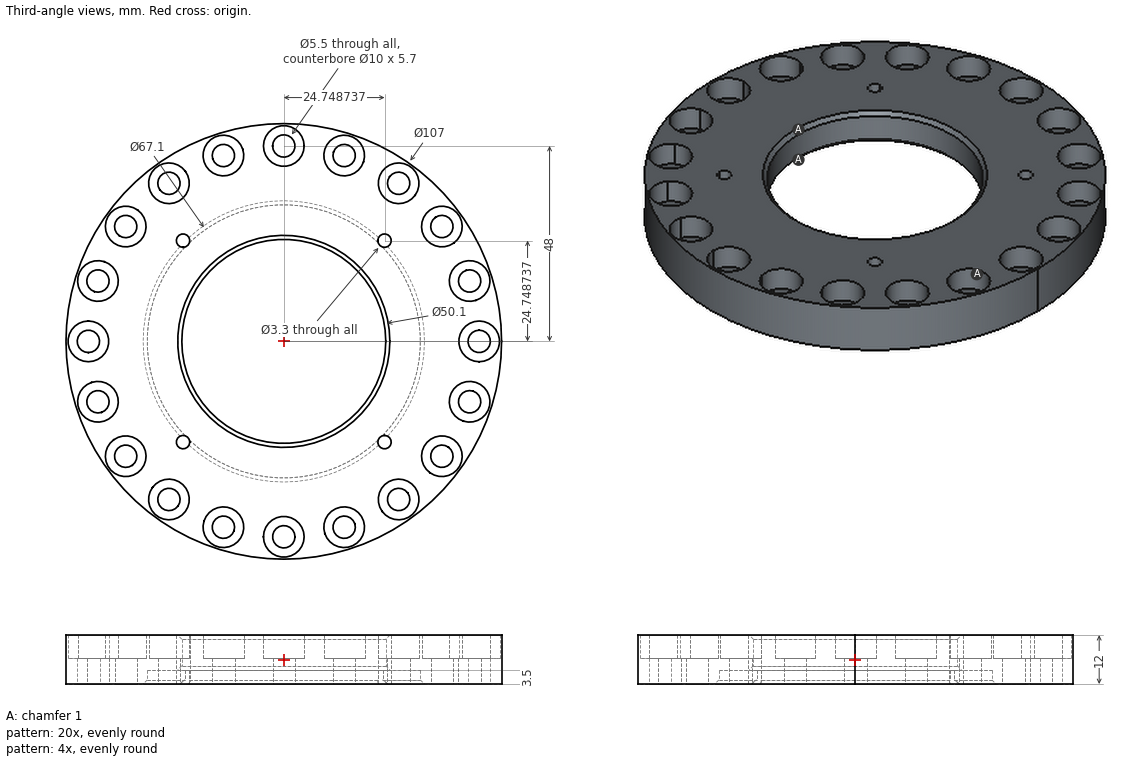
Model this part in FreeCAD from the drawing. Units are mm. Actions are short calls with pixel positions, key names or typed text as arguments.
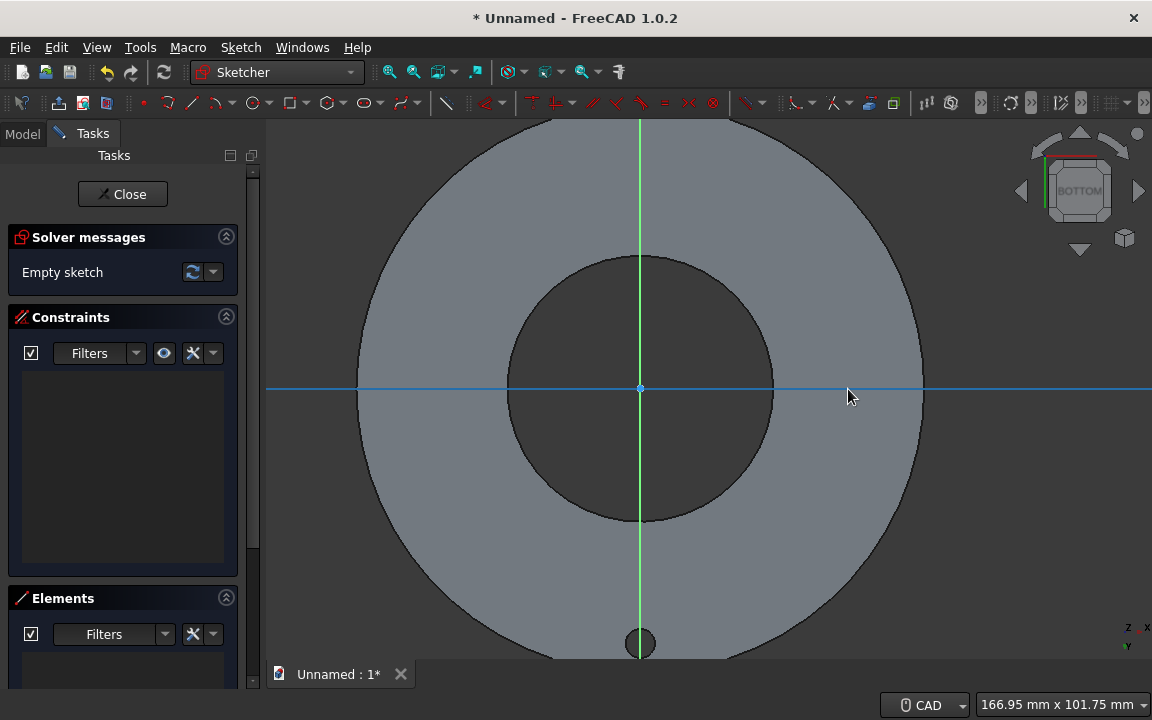
click(254, 104)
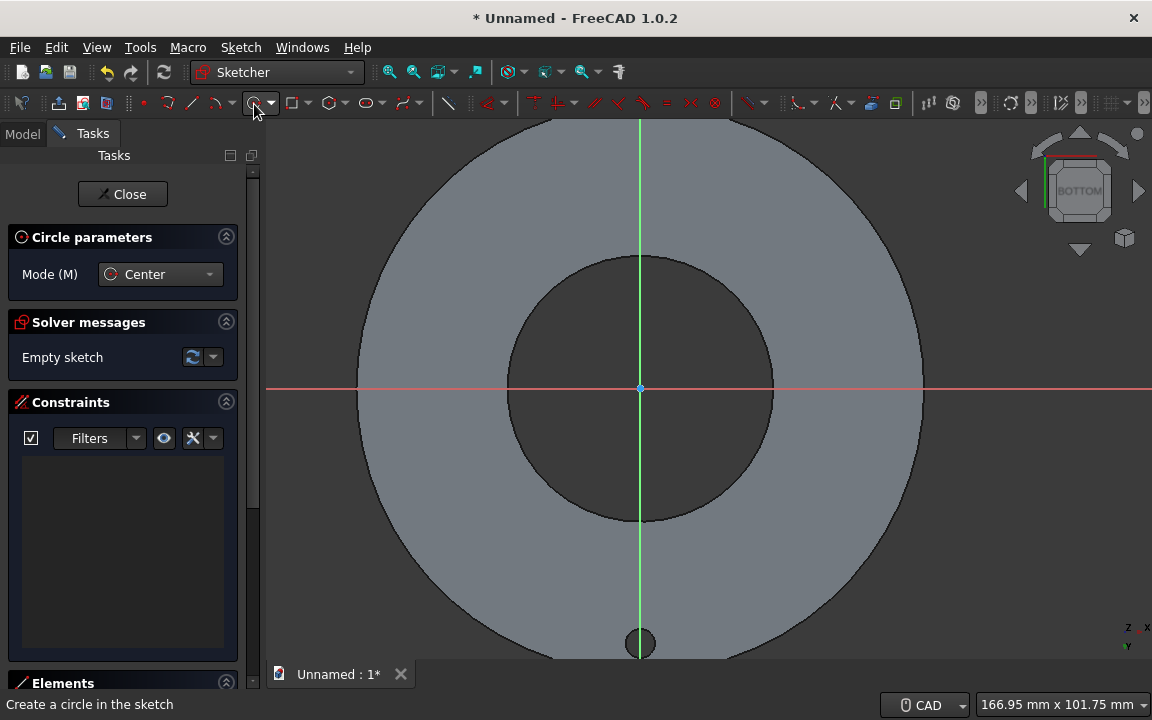
click(640, 389)
click(766, 263)
key(Escape)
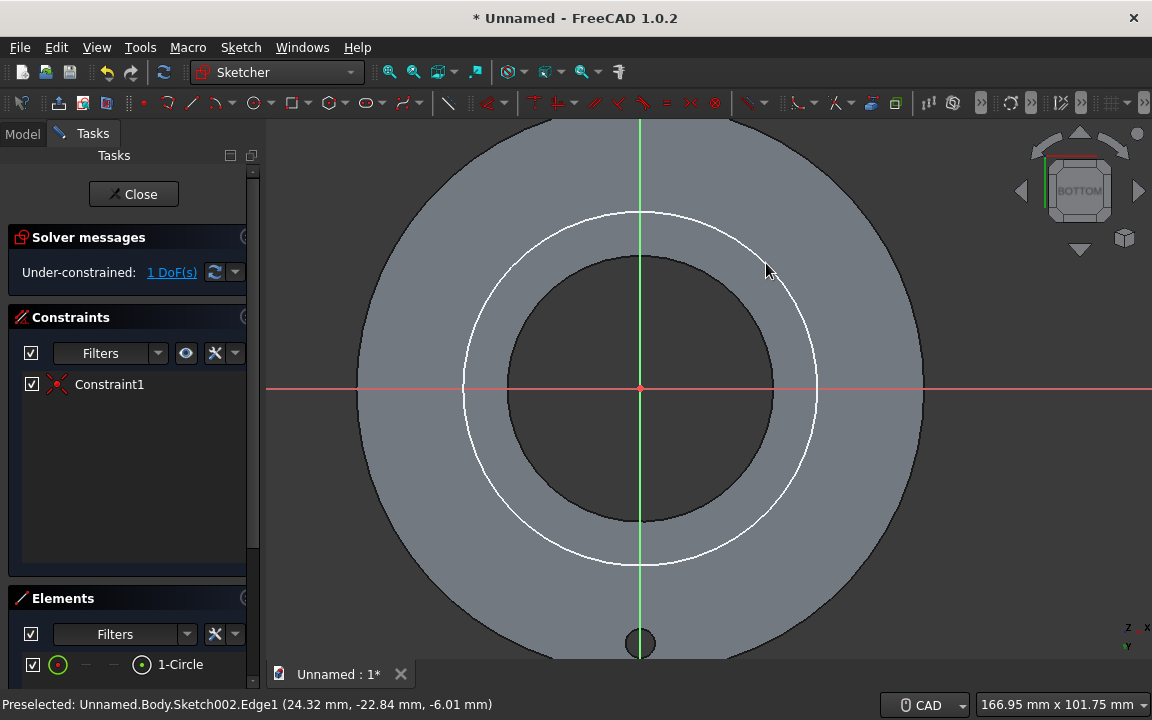
click(488, 104)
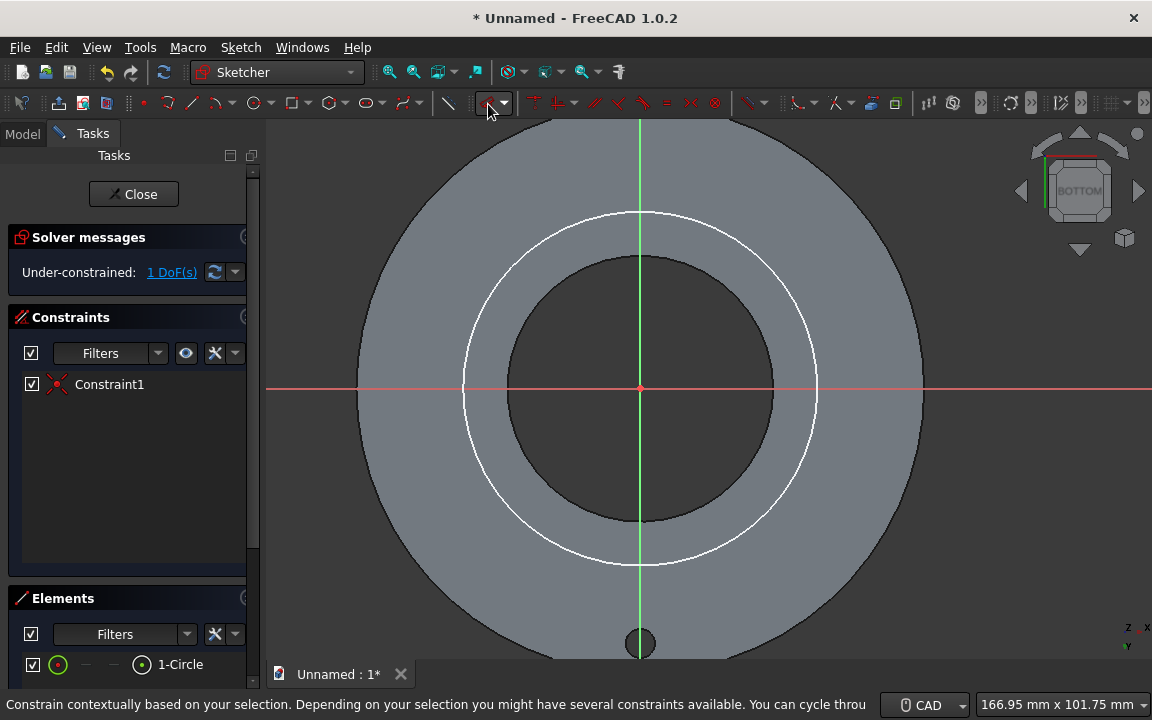
click(765, 263)
click(788, 240)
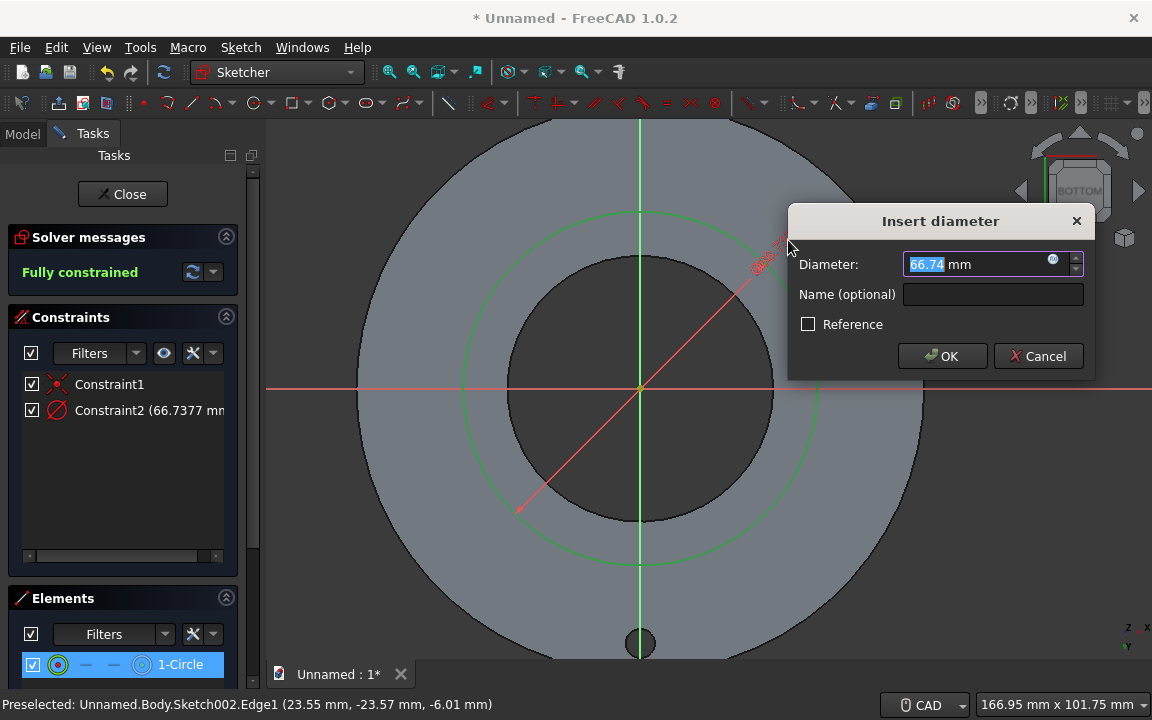
text(67.1)
key(Return)
key(Escape)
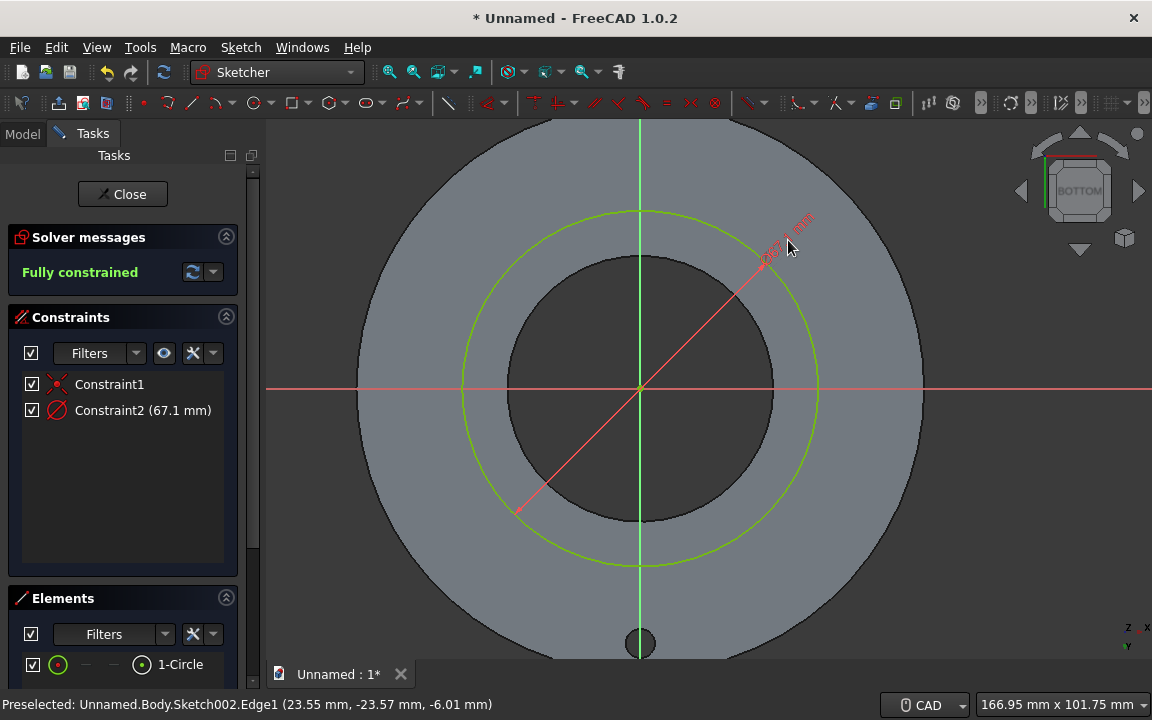
click(123, 194)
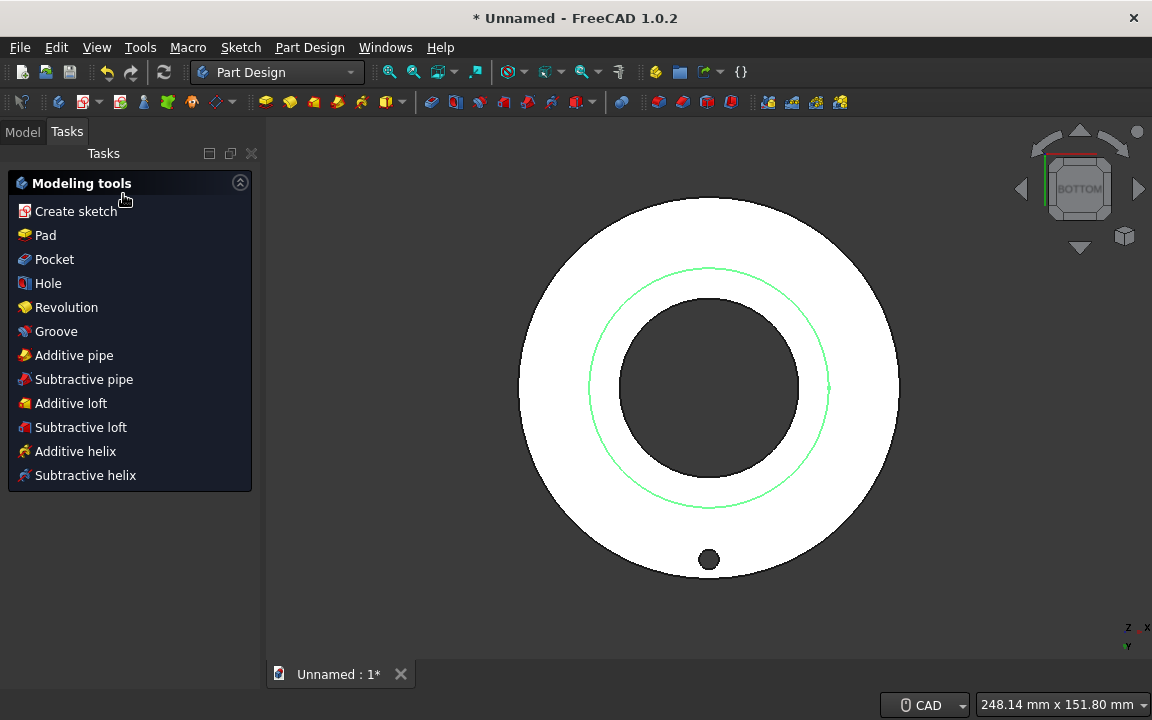
click(432, 102)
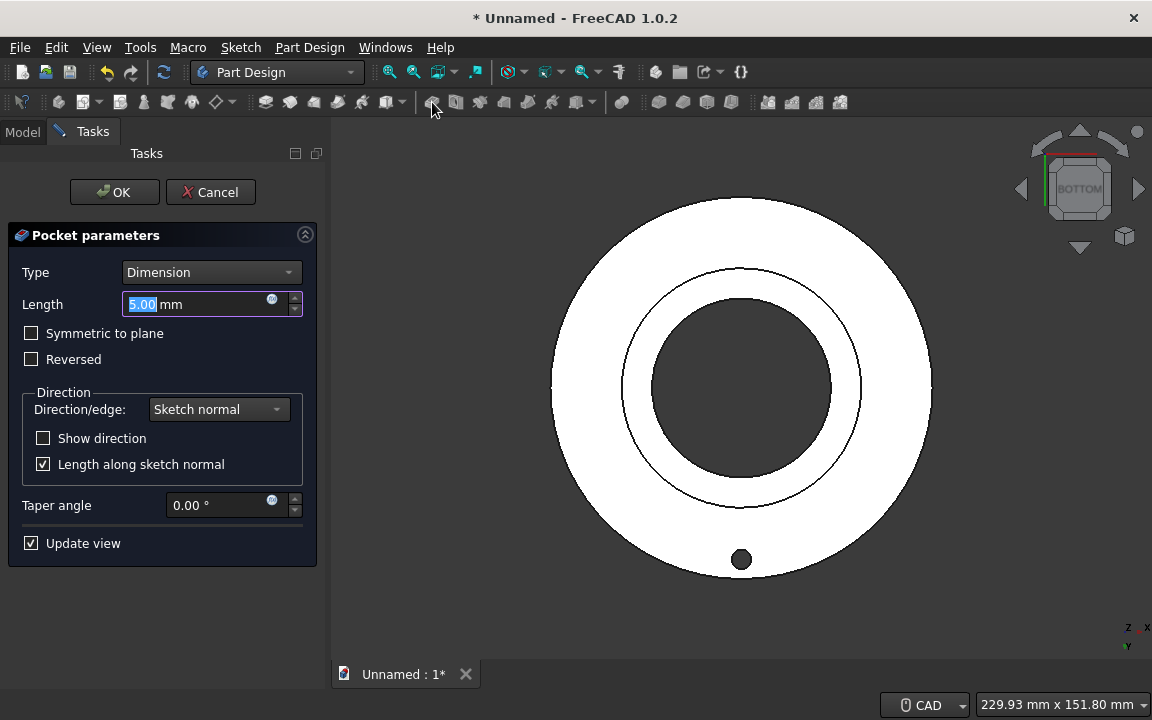
text(3.5)
key(Tab)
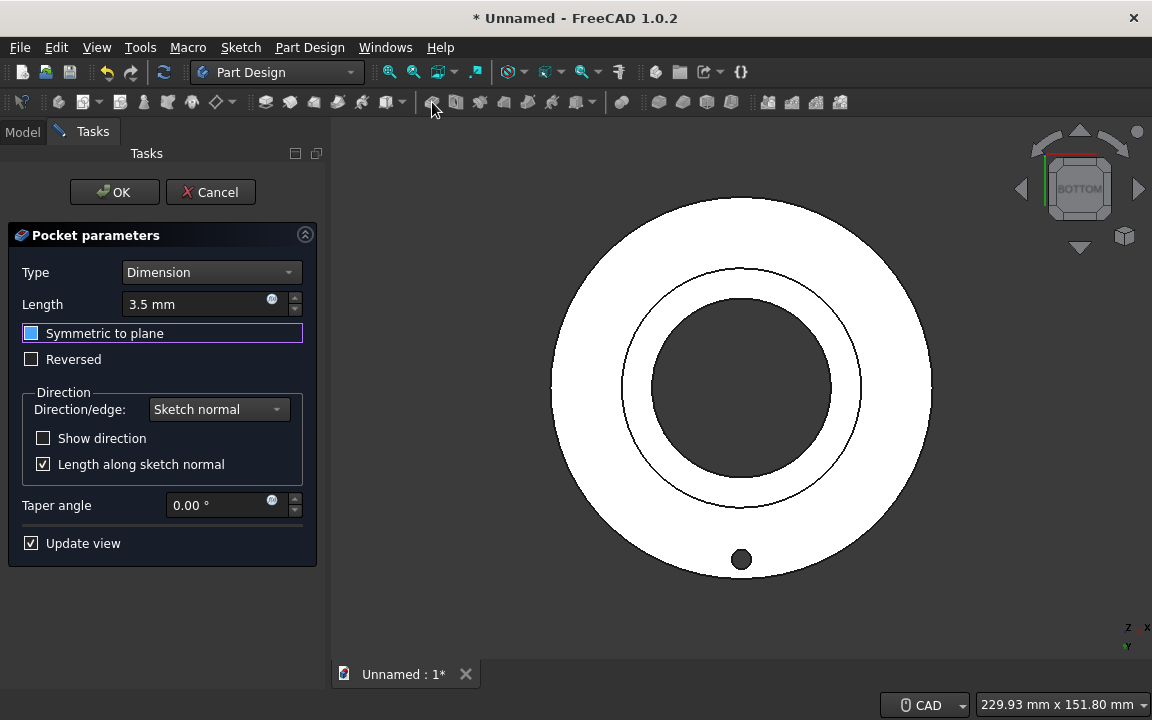
click(115, 192)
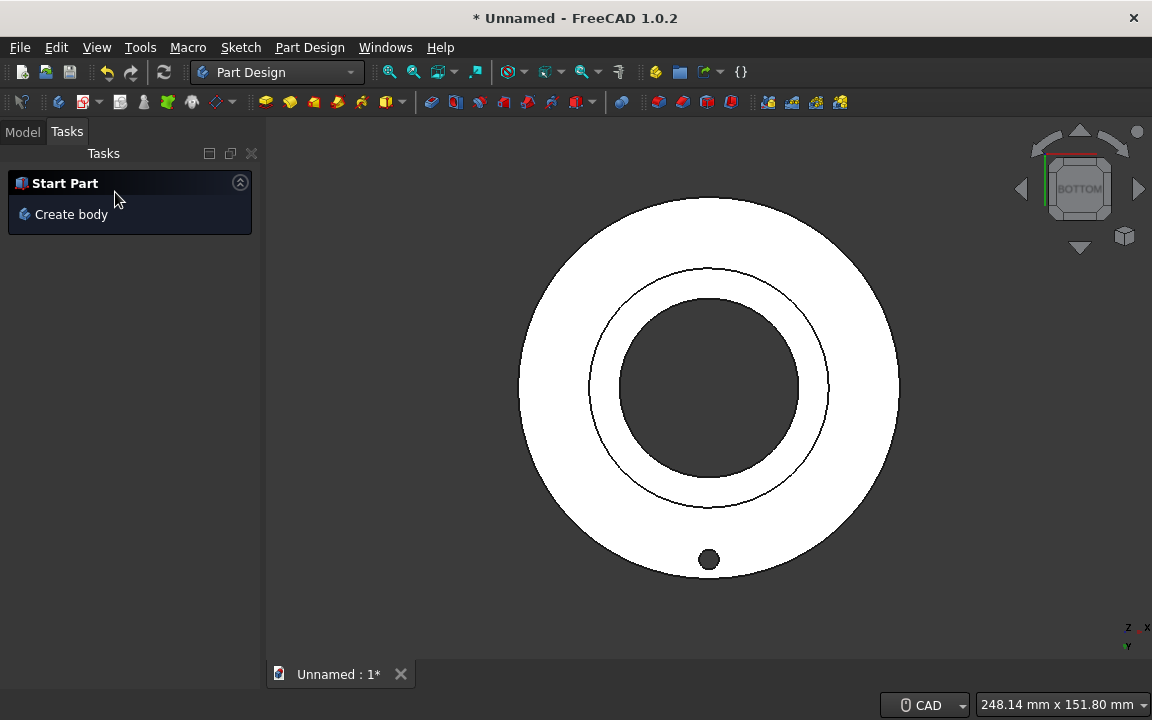
click(620, 387)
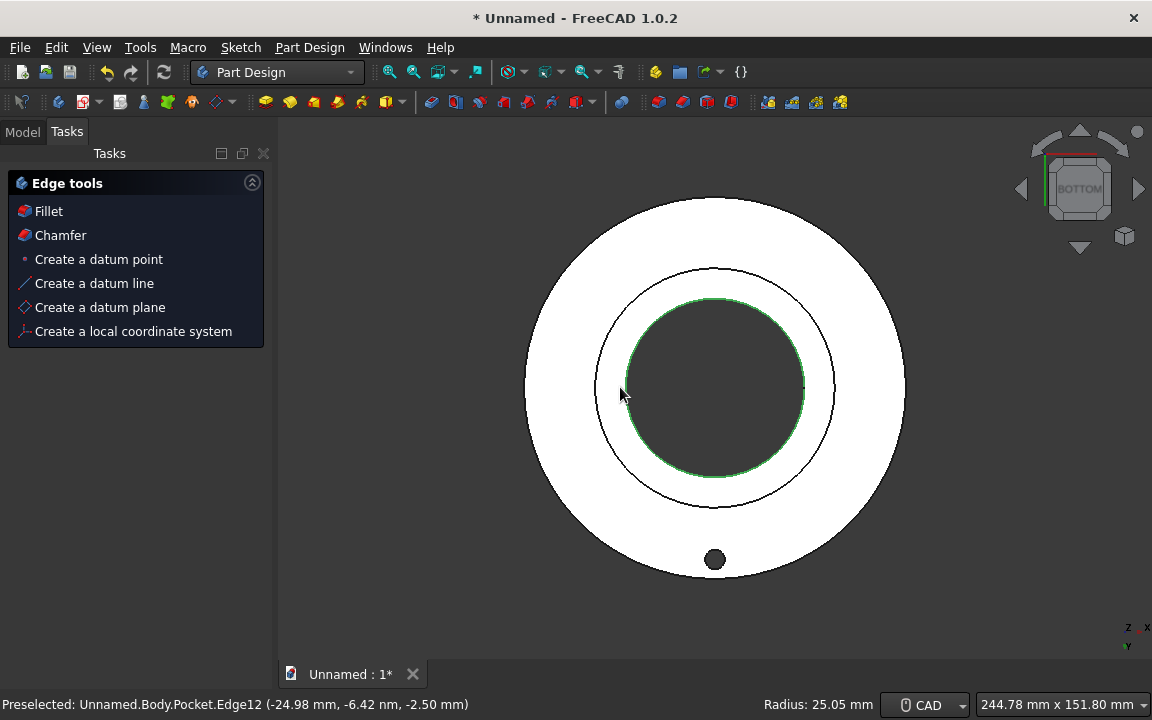
click(595, 387, ctrl)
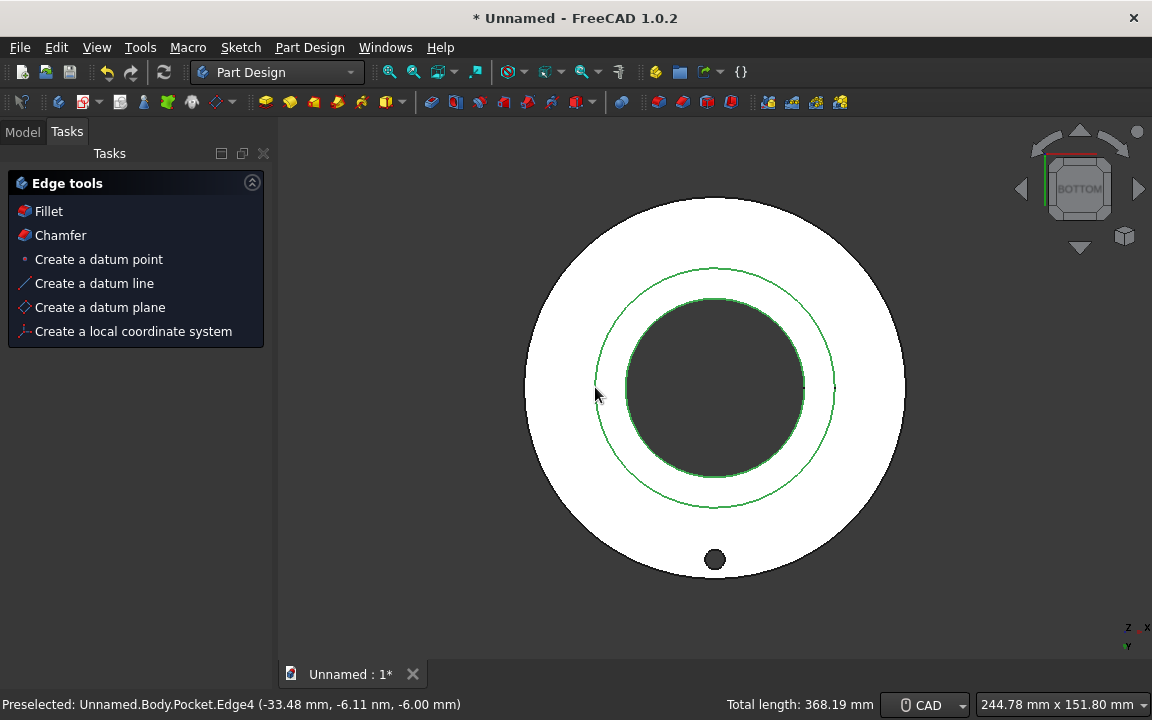
key(0)